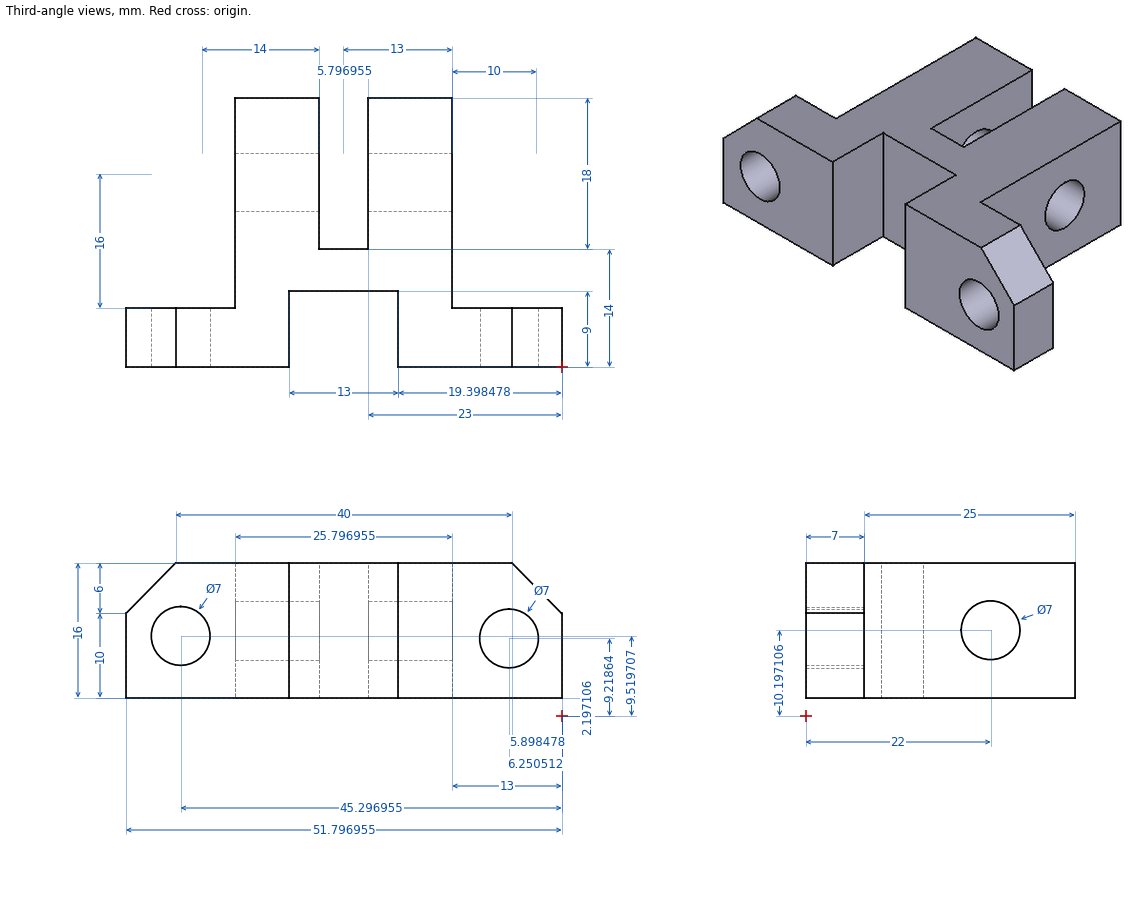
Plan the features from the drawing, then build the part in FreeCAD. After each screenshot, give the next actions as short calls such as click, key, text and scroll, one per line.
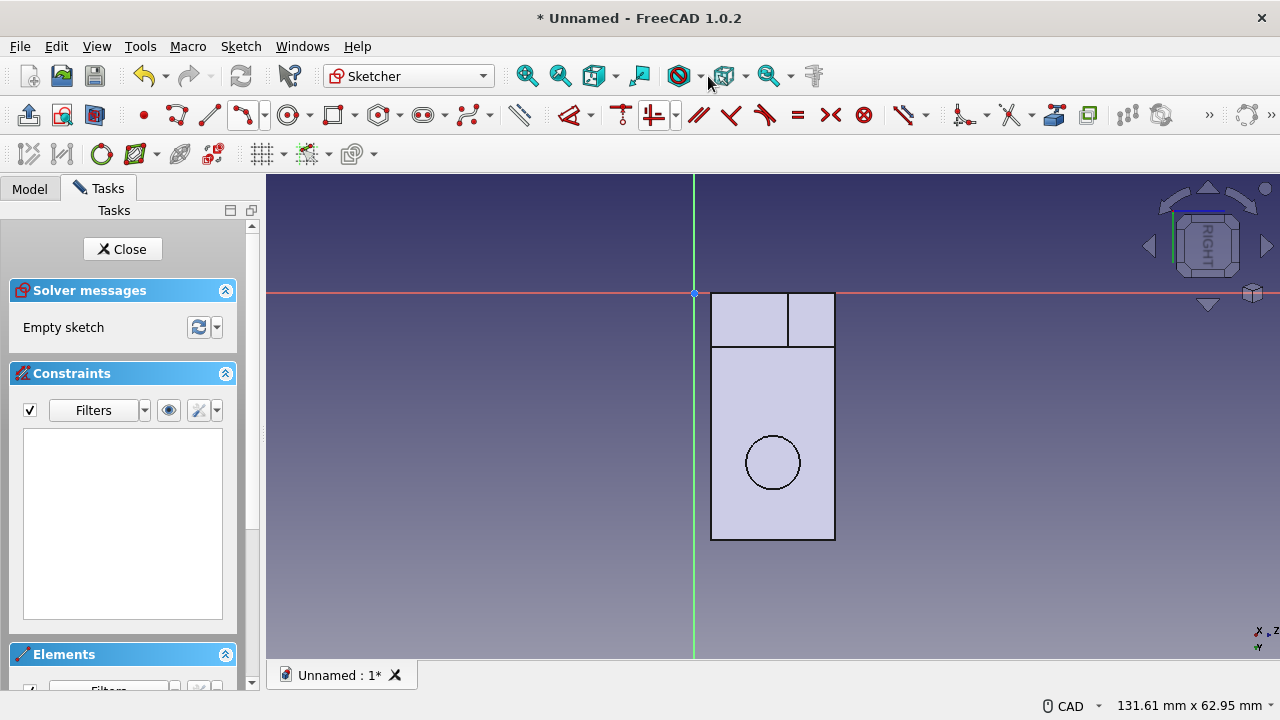
scroll(787, 472, up, 9)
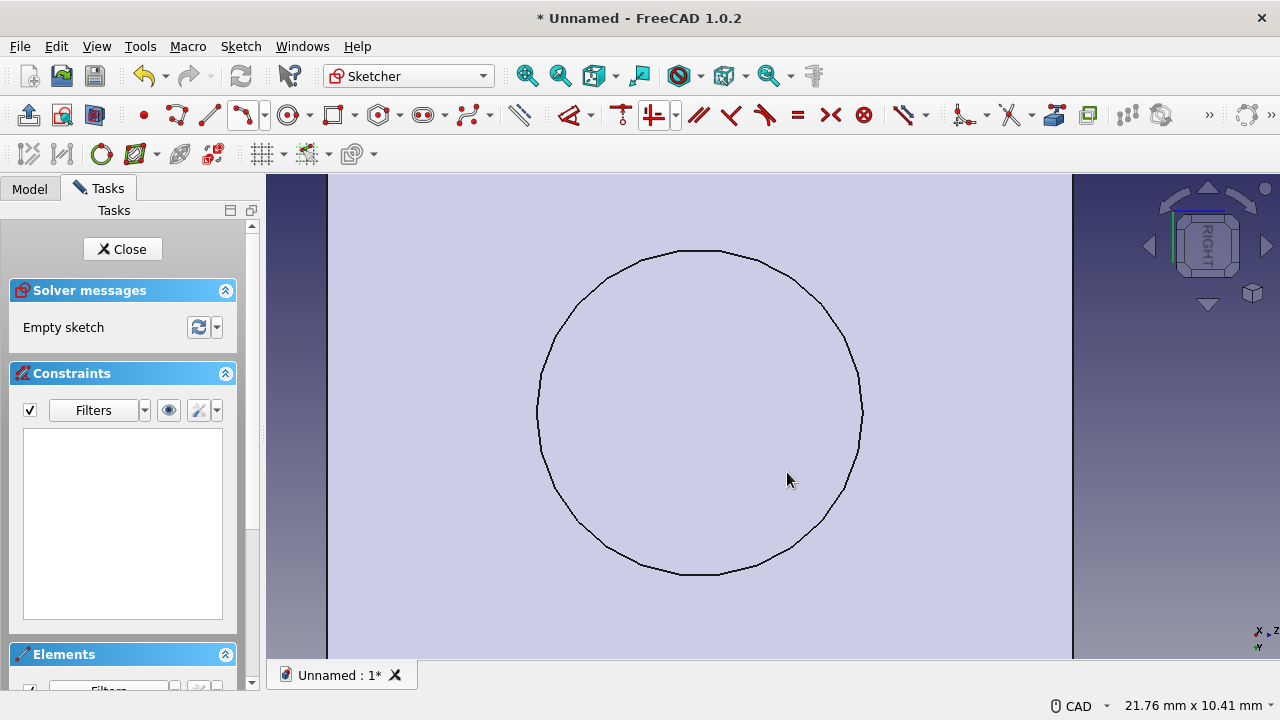
click(288, 116)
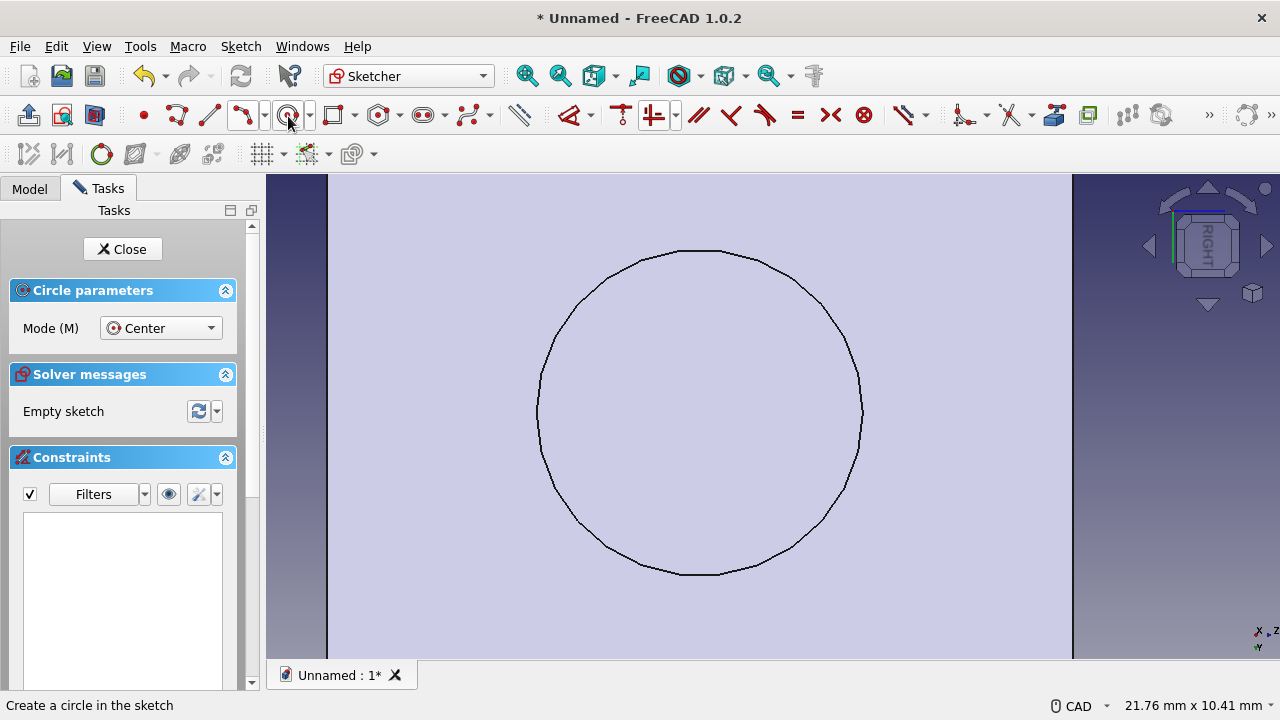
click(700, 413)
click(815, 297)
key(Escape)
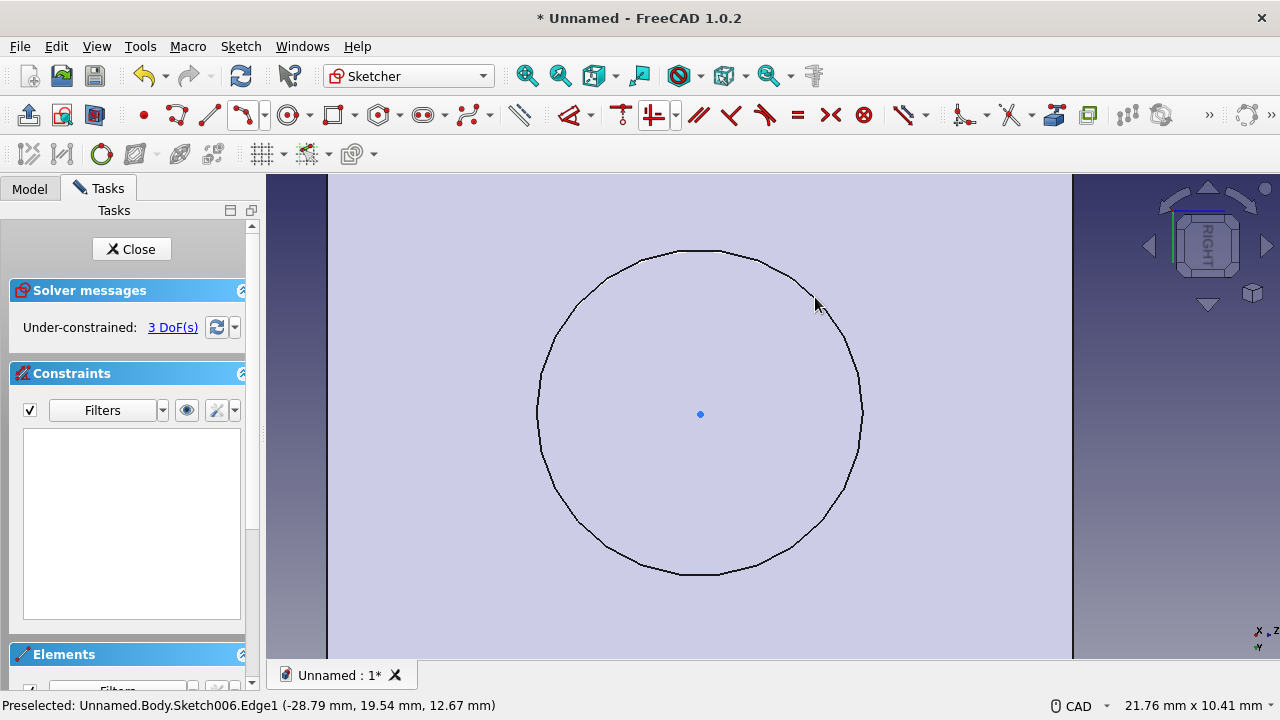
click(568, 116)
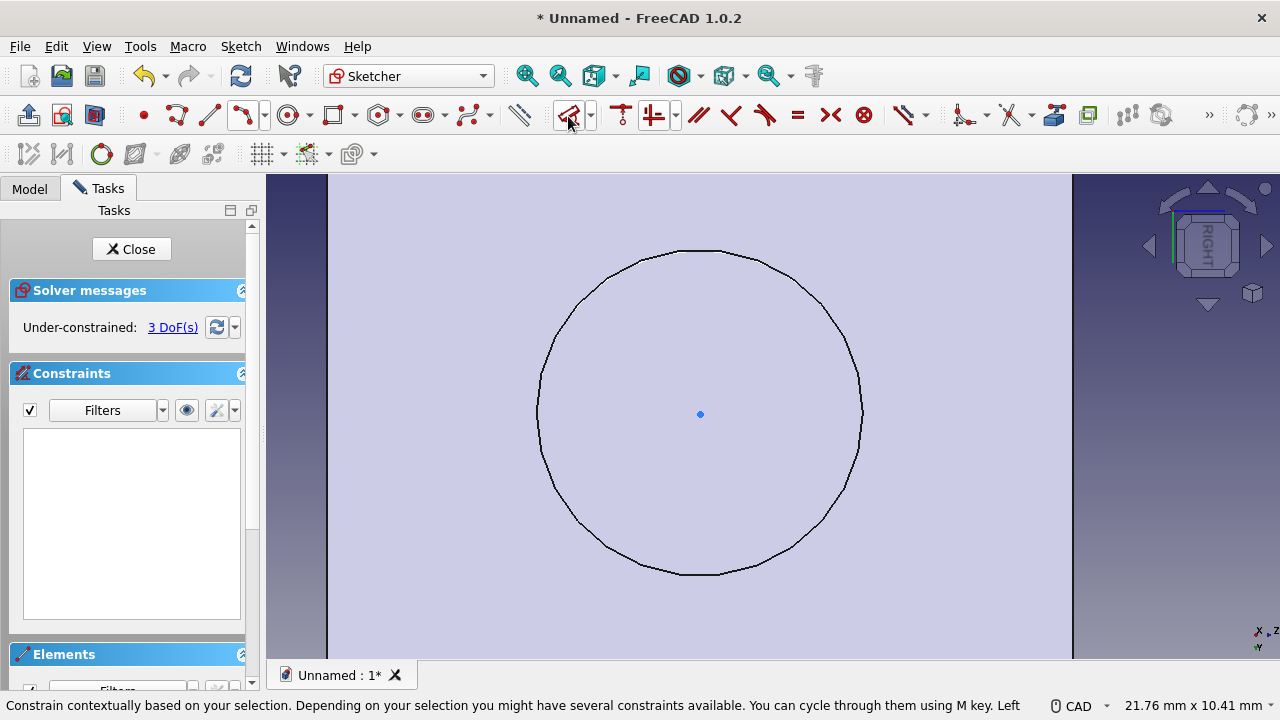
click(815, 298)
click(838, 275)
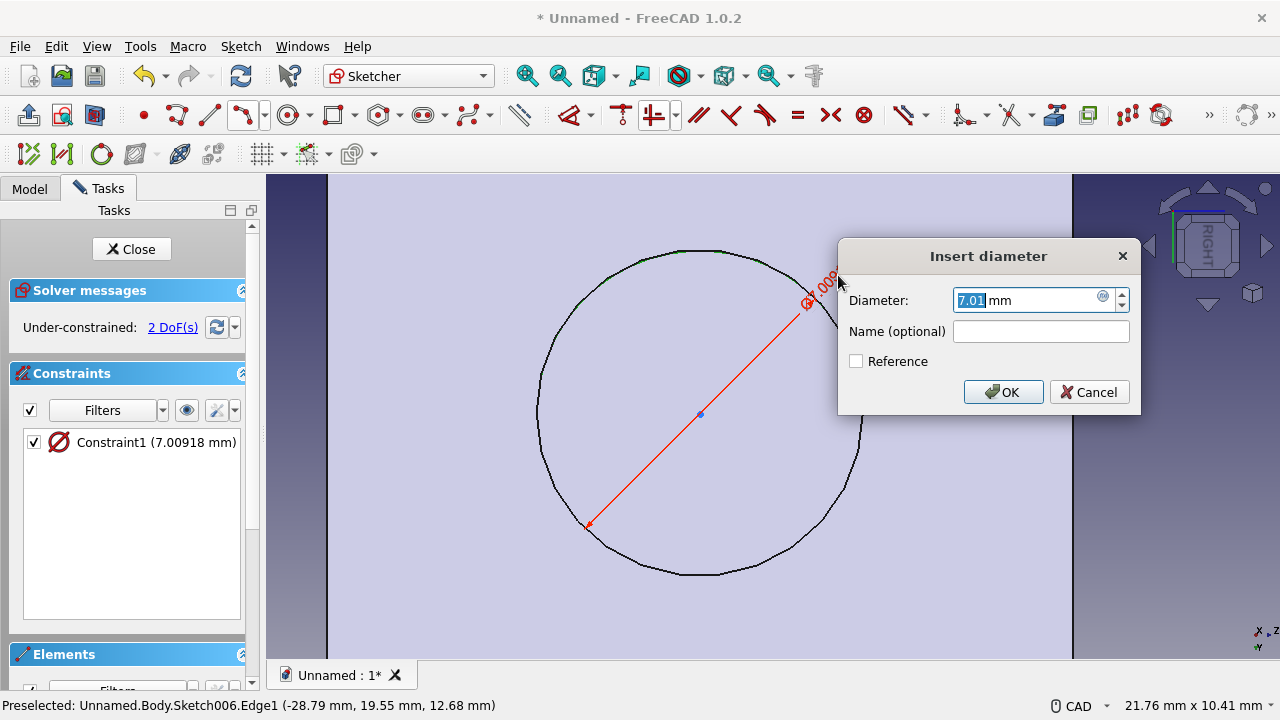
text(7)
key(Return)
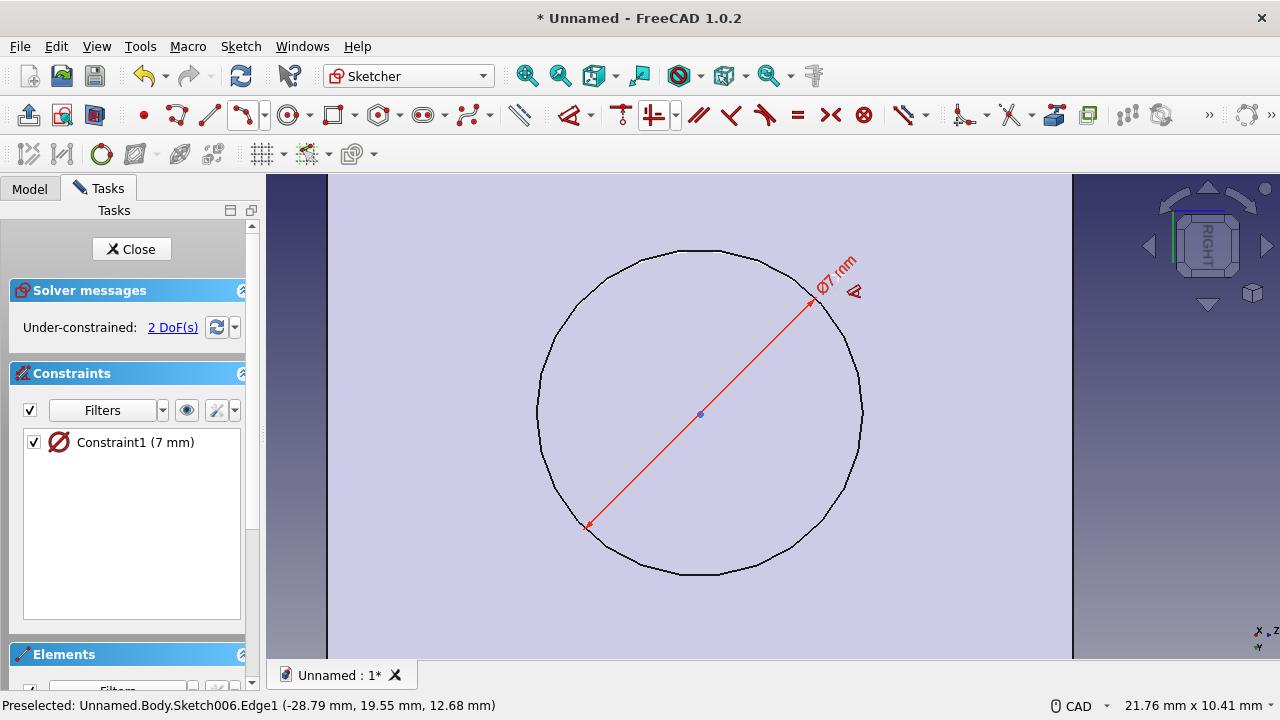
click(700, 414)
click(734, 308)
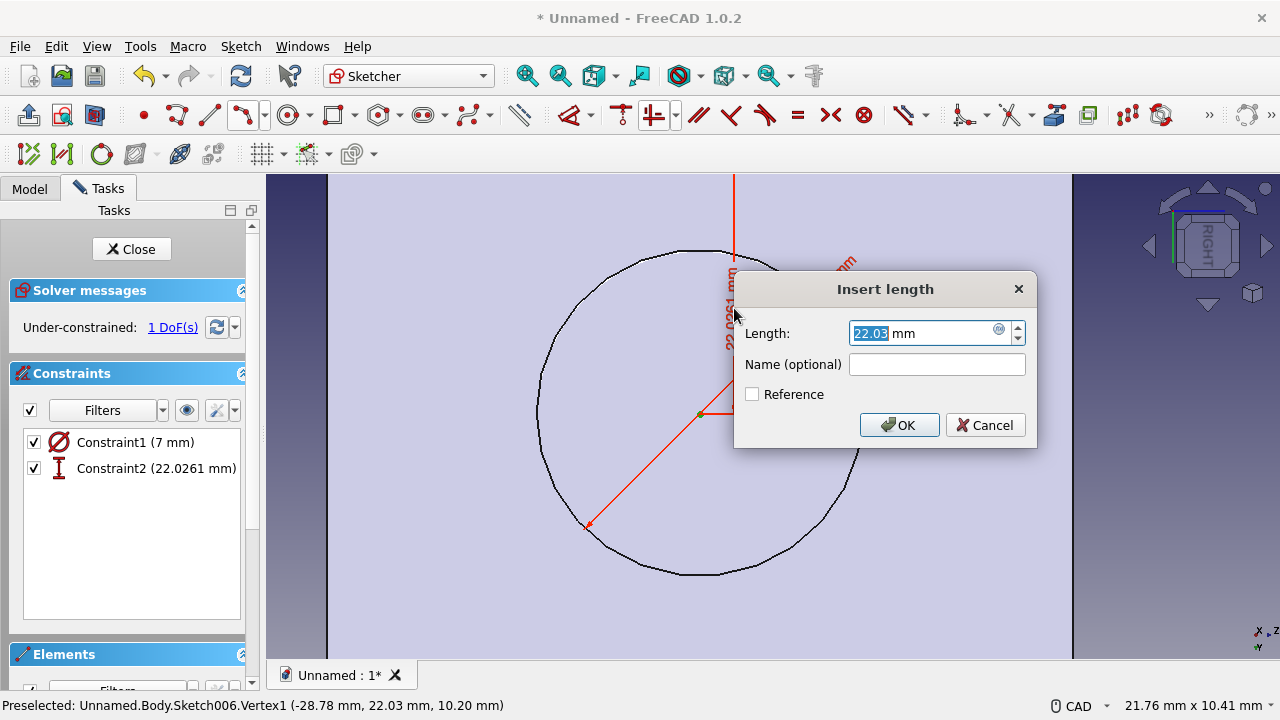
text(22)
key(Return)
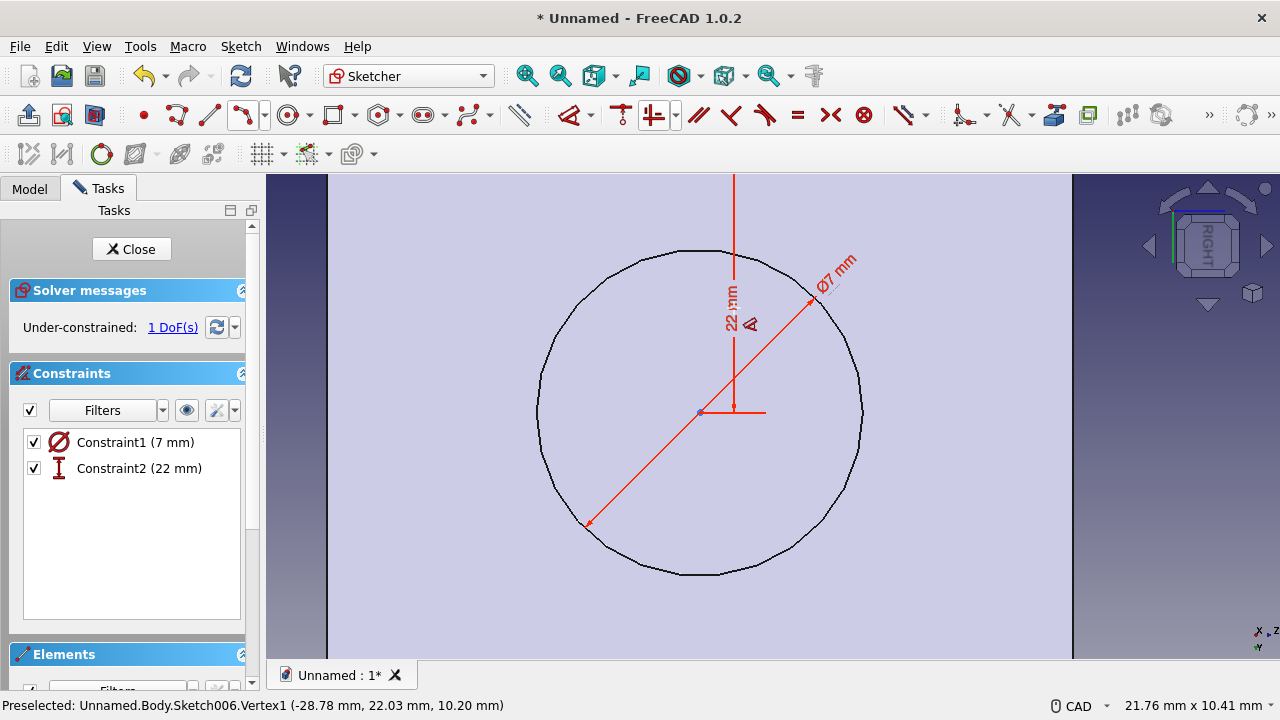
click(700, 413)
click(497, 447)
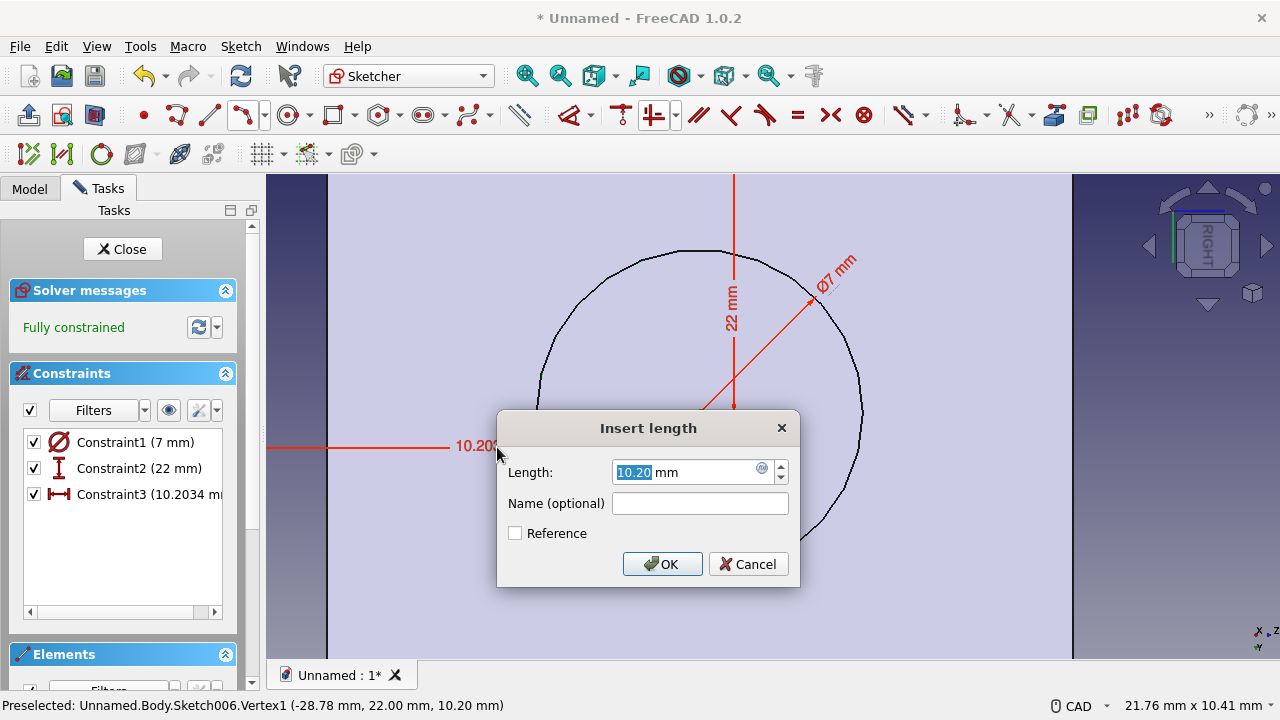
text(10.197106)
key(Return)
key(Escape)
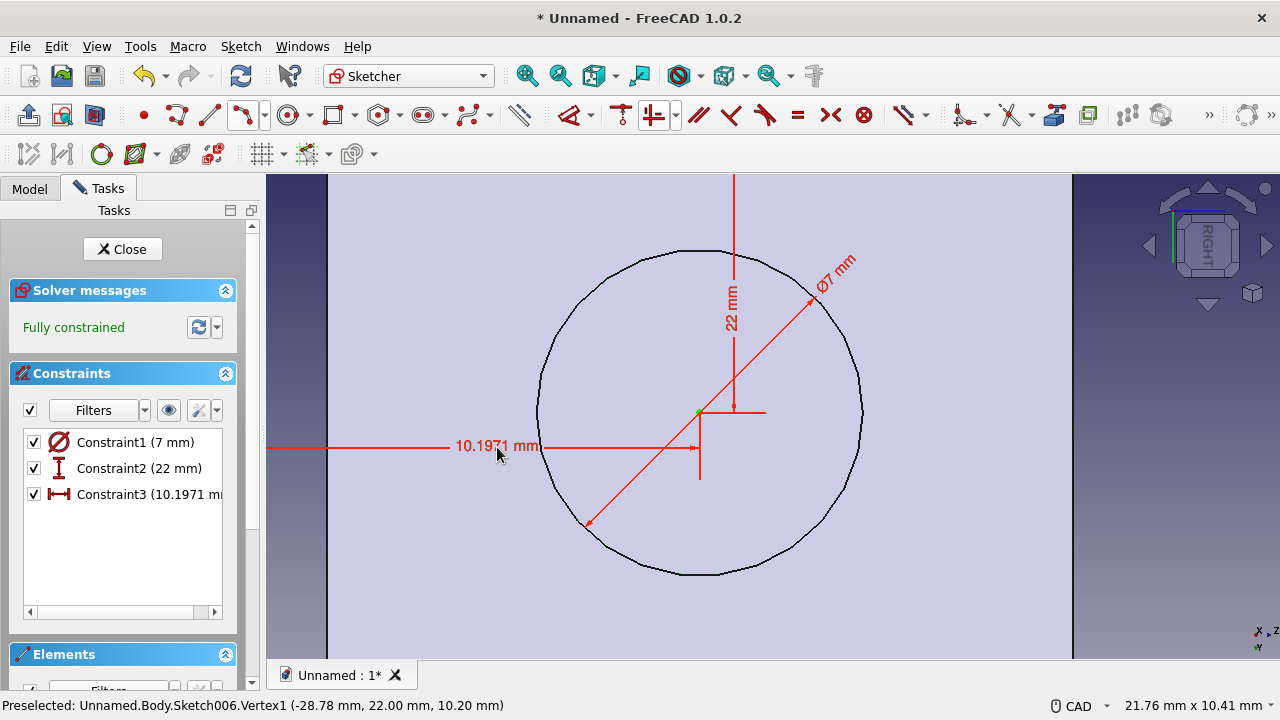
click(123, 249)